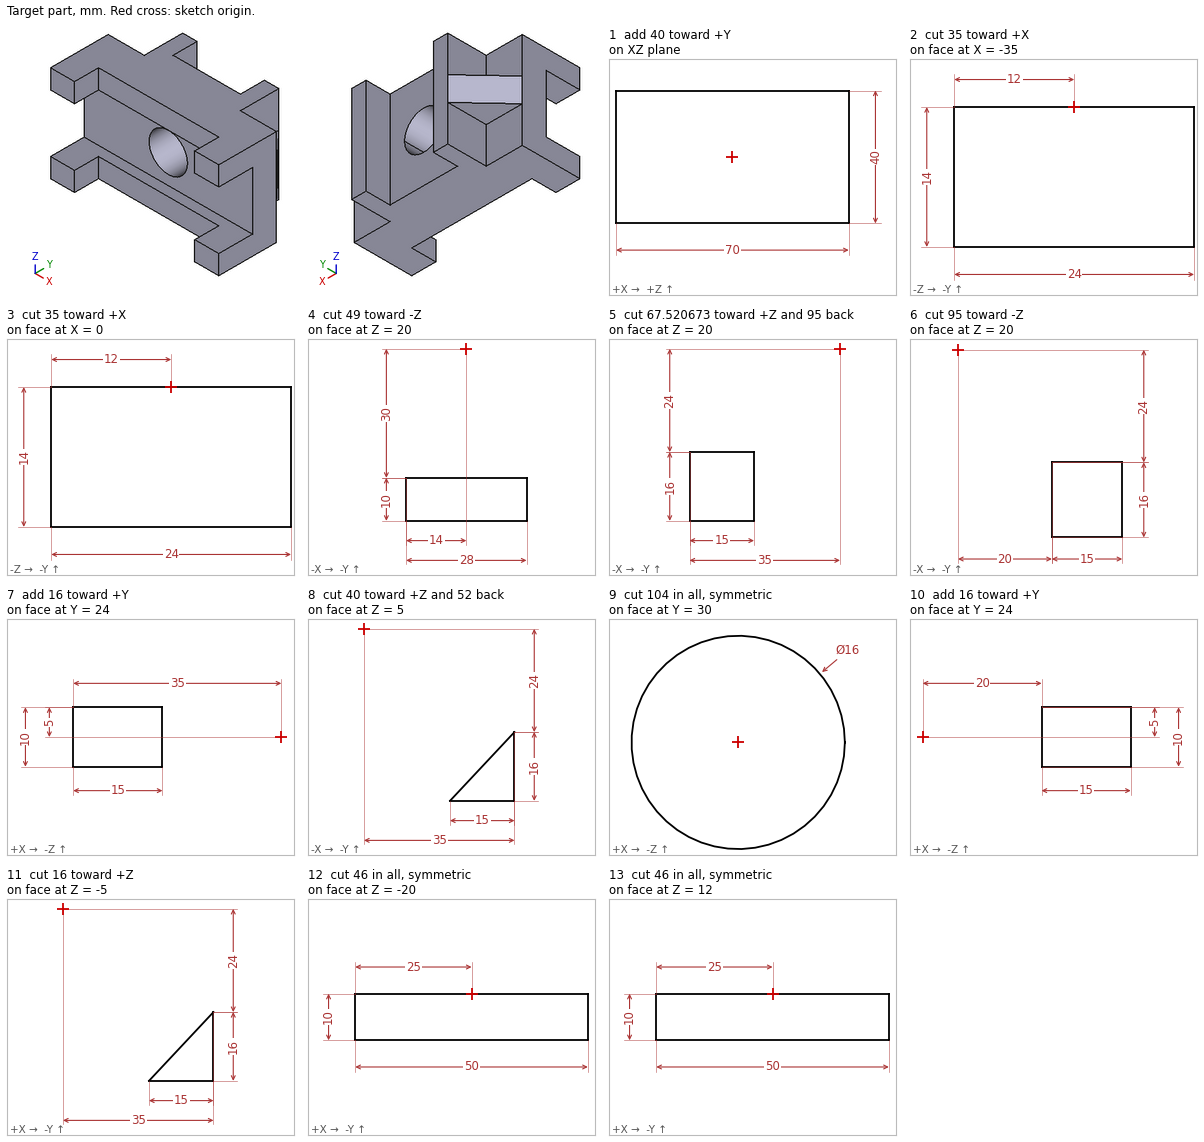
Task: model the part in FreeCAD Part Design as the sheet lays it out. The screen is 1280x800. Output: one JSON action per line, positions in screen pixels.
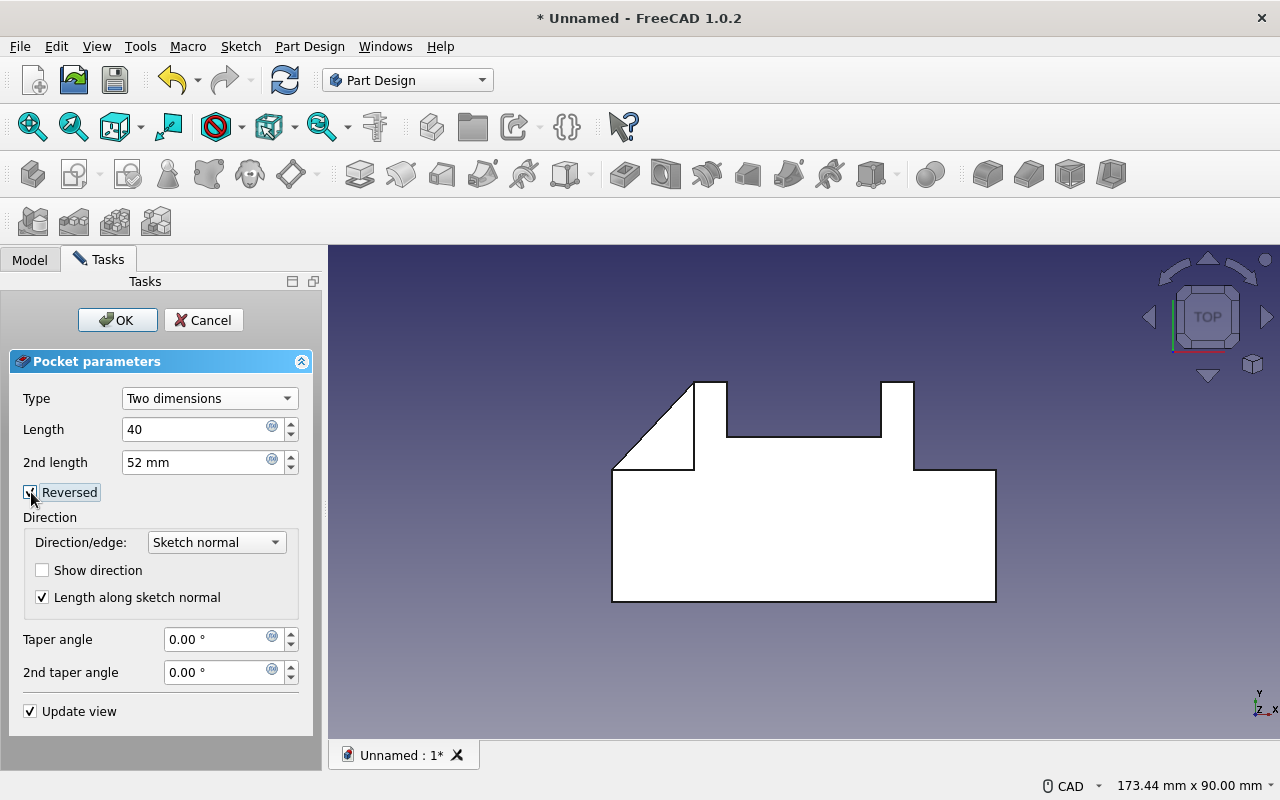
{"action": "left_click", "coordinate": [118, 320]}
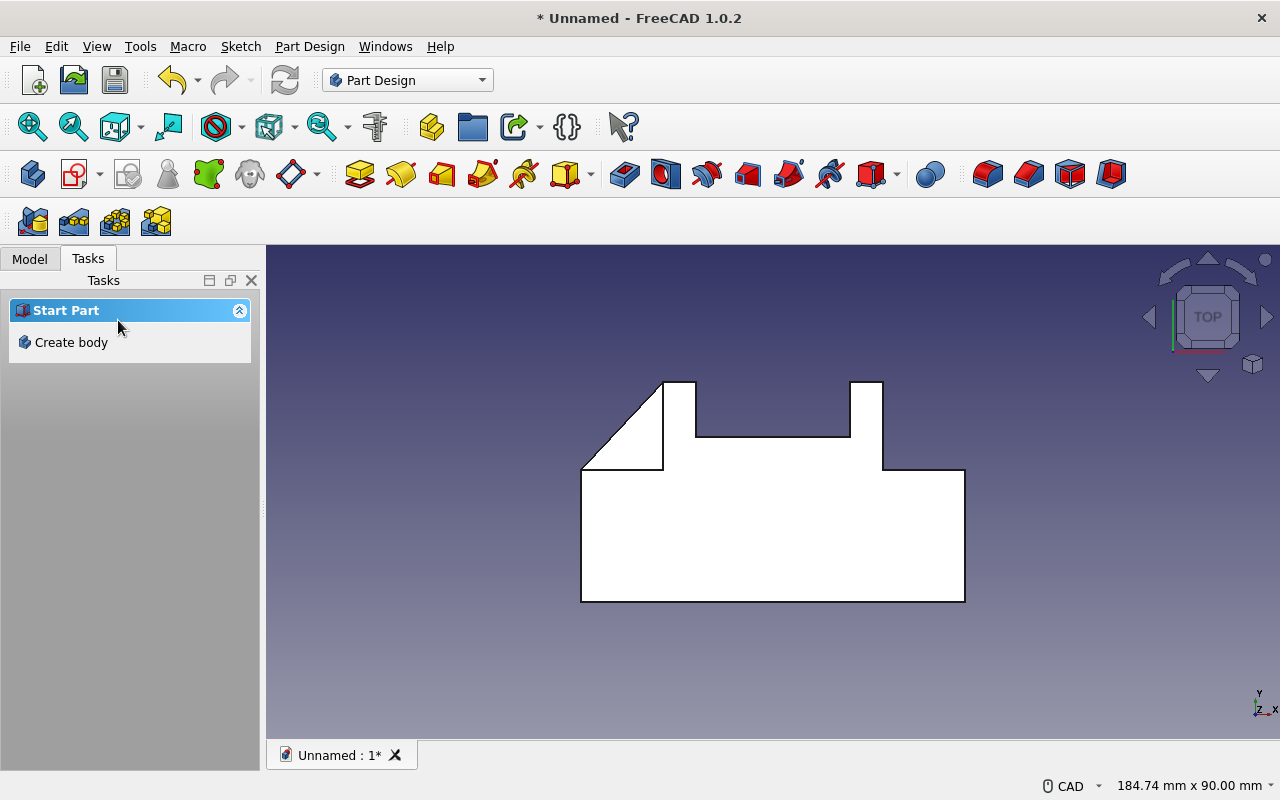
{"action": "key", "text": "v f"}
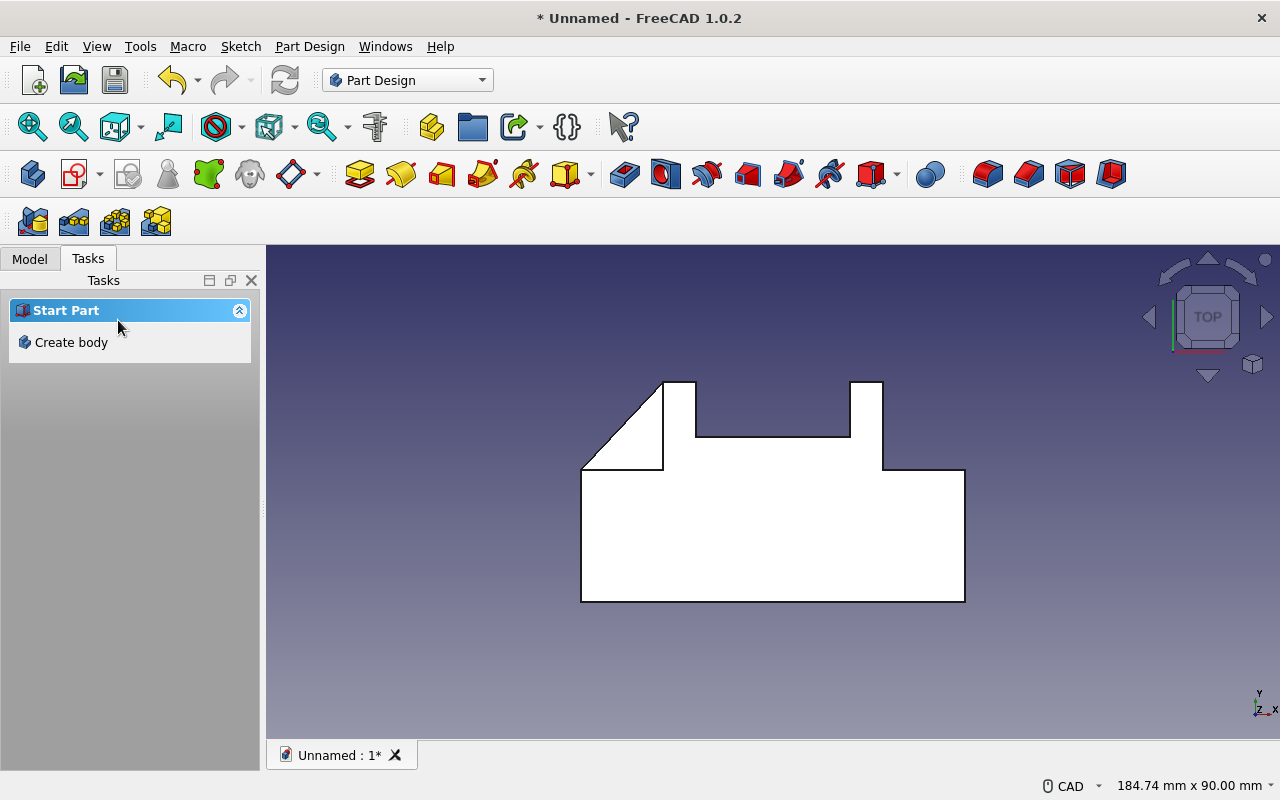
{"action": "key", "text": "4"}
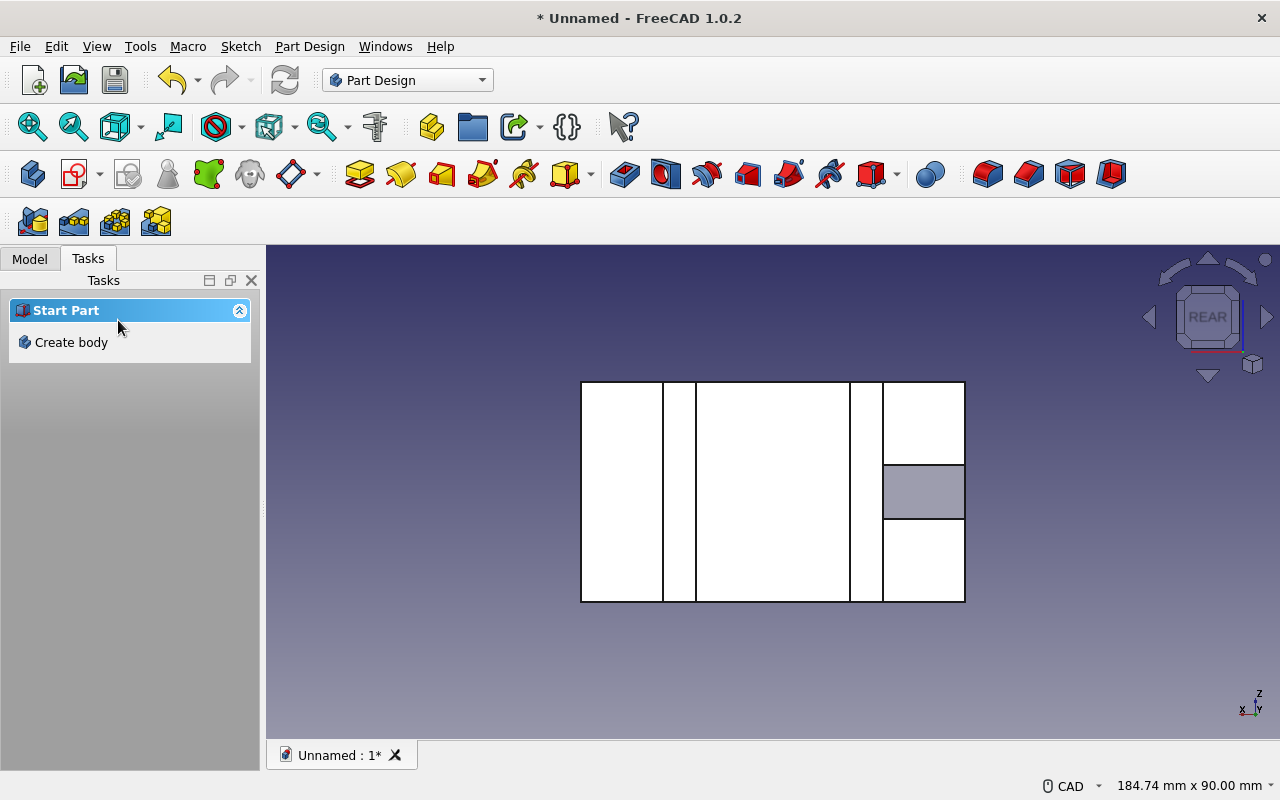
{"action": "key", "text": "v f"}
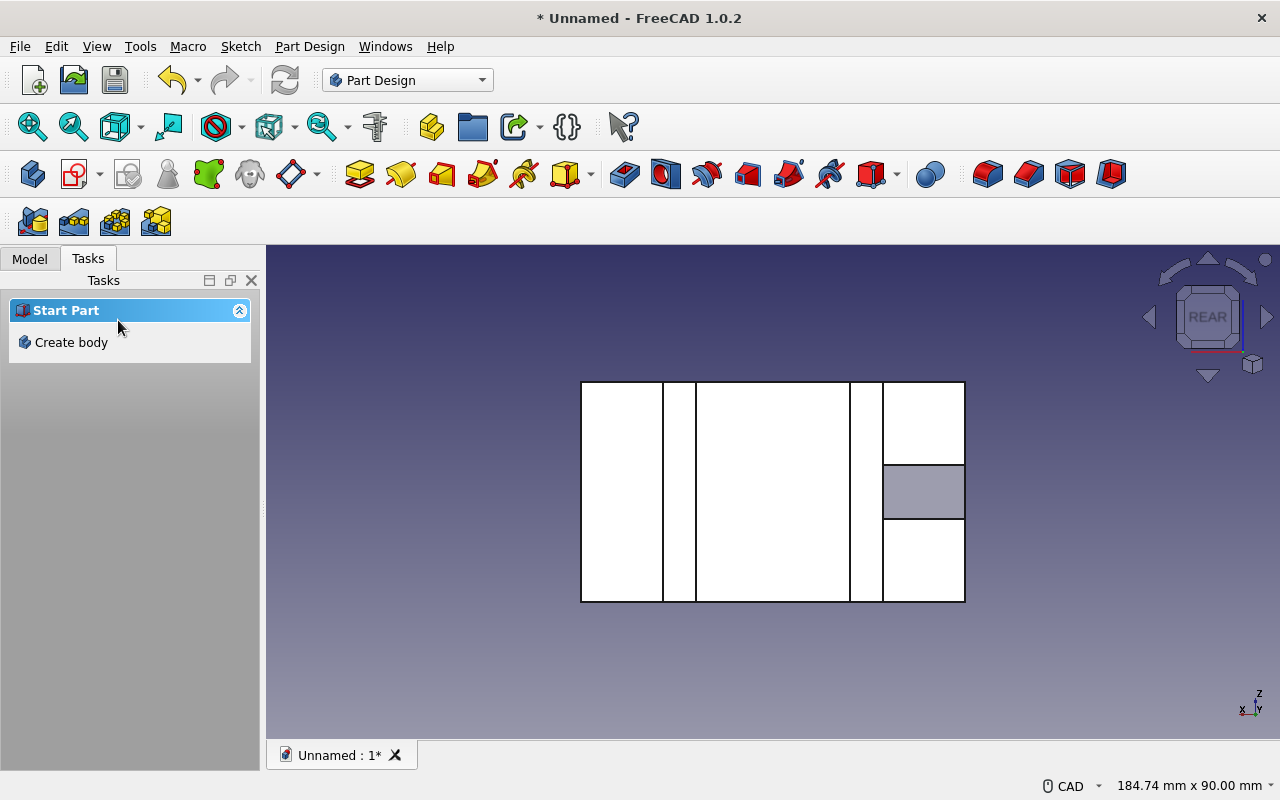
{"action": "left_click", "coordinate": [773, 460]}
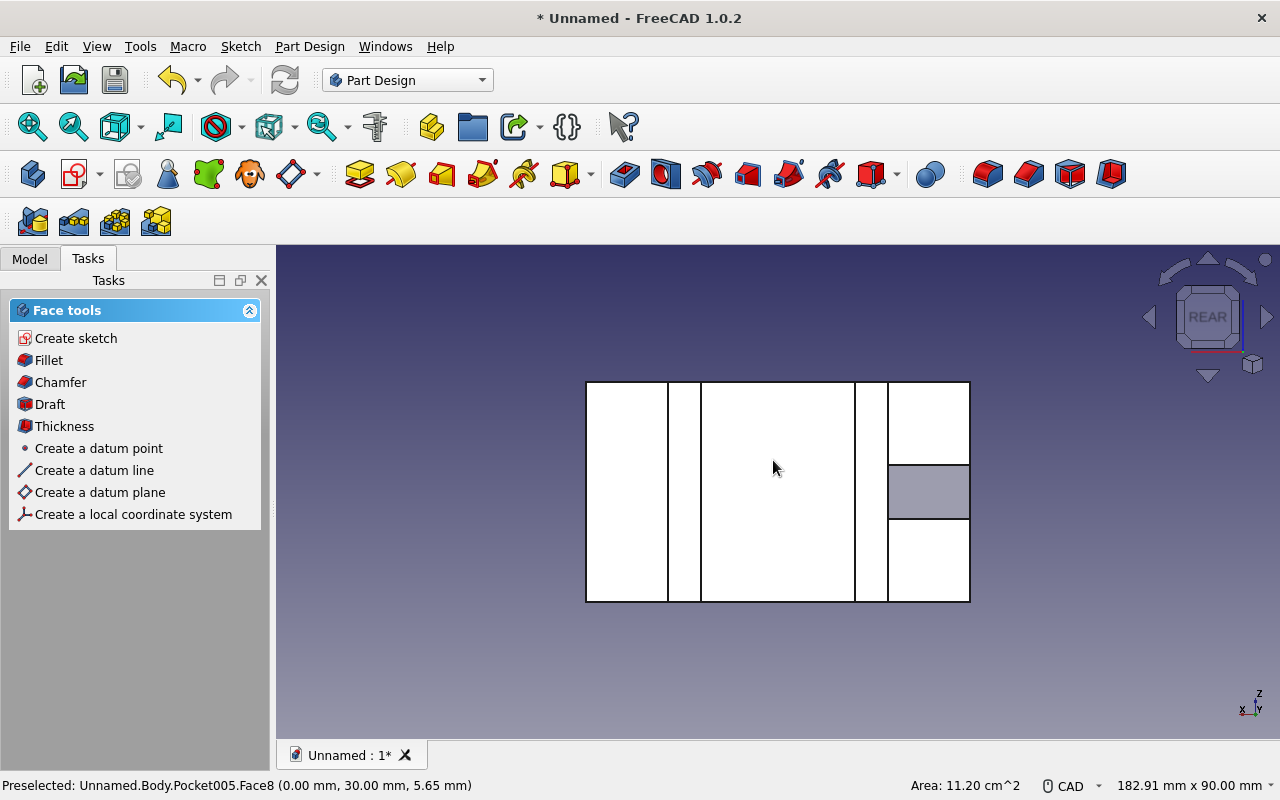
{"action": "left_click", "coordinate": [74, 174]}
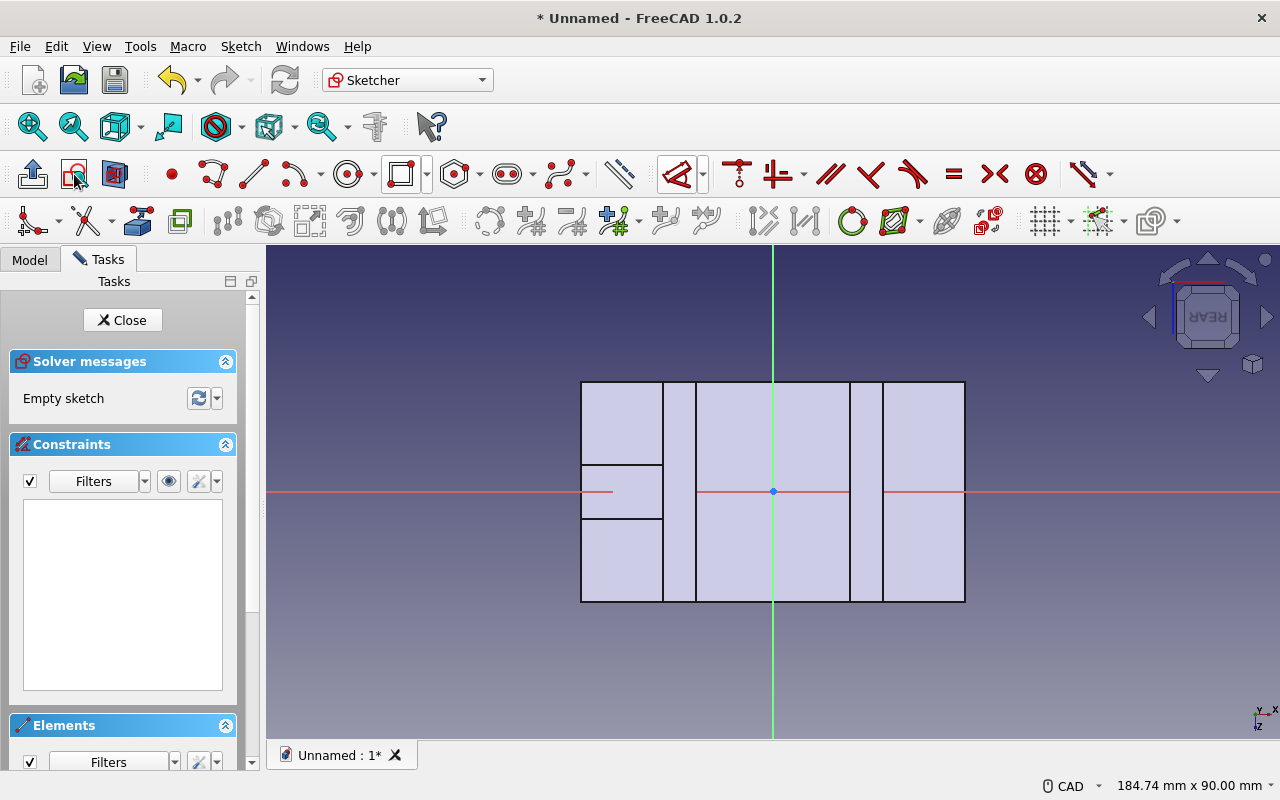
{"action": "left_click", "coordinate": [115, 174]}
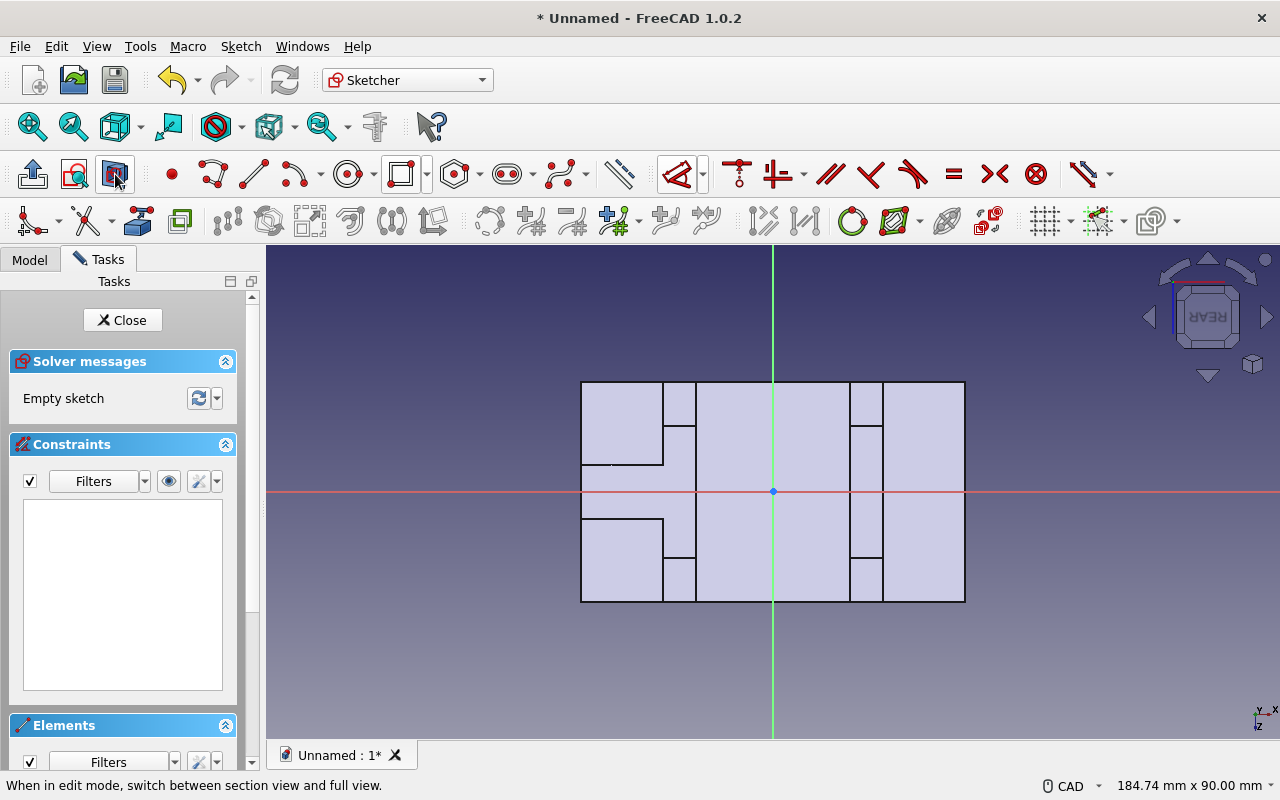
{"action": "scroll", "coordinate": [803, 492], "scroll_direction": "up", "scroll_amount": 6}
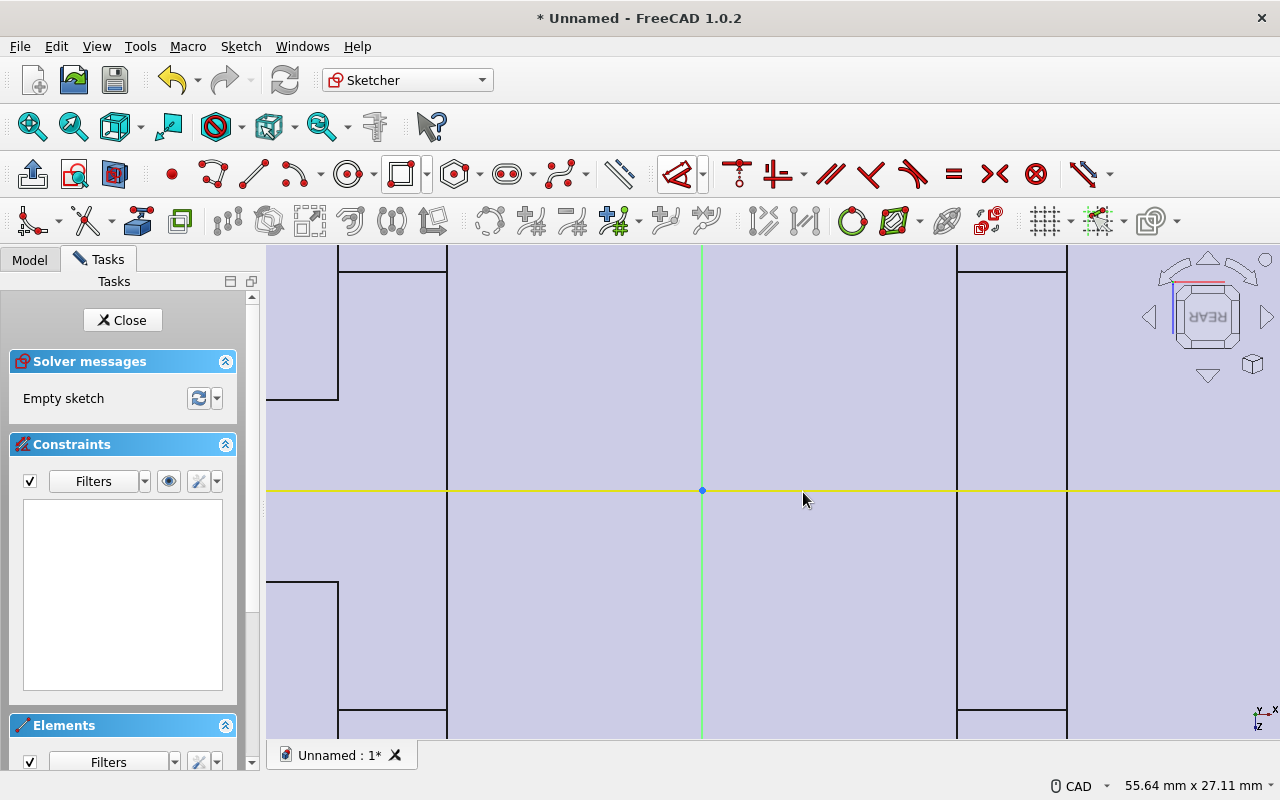
{"action": "key", "text": "g c"}